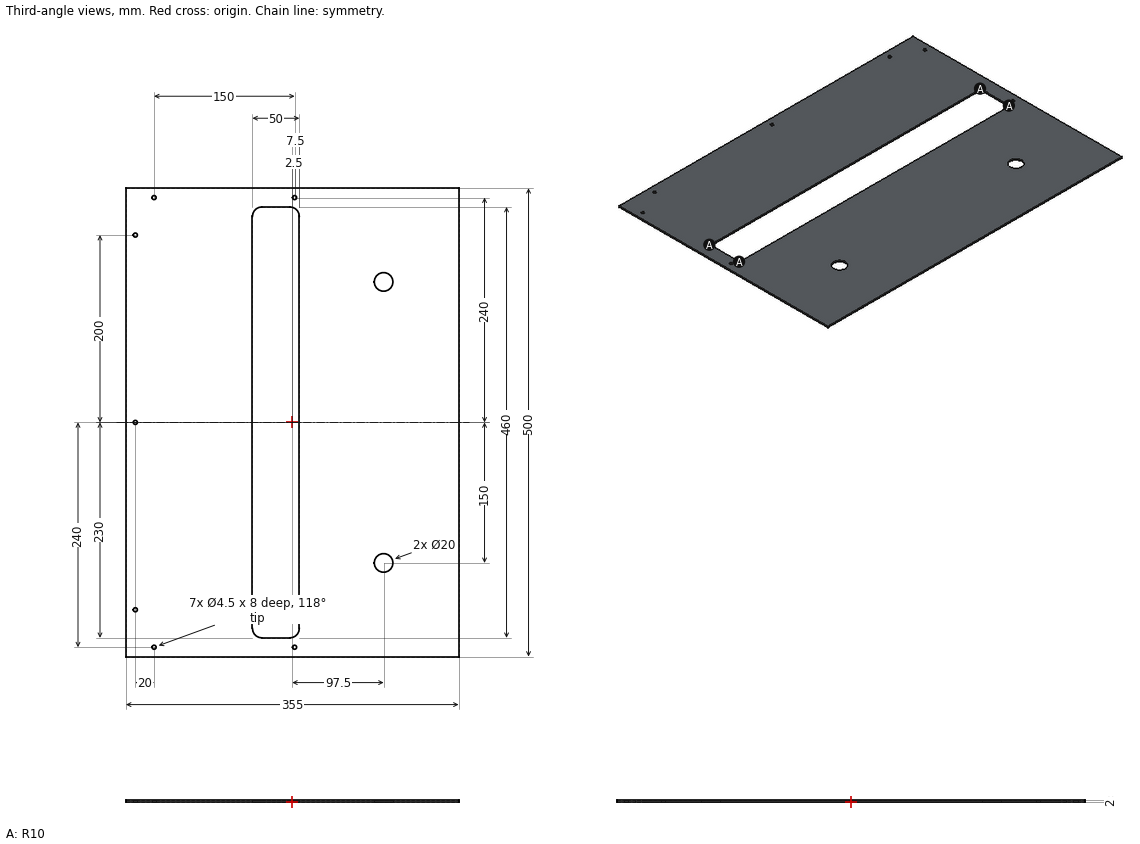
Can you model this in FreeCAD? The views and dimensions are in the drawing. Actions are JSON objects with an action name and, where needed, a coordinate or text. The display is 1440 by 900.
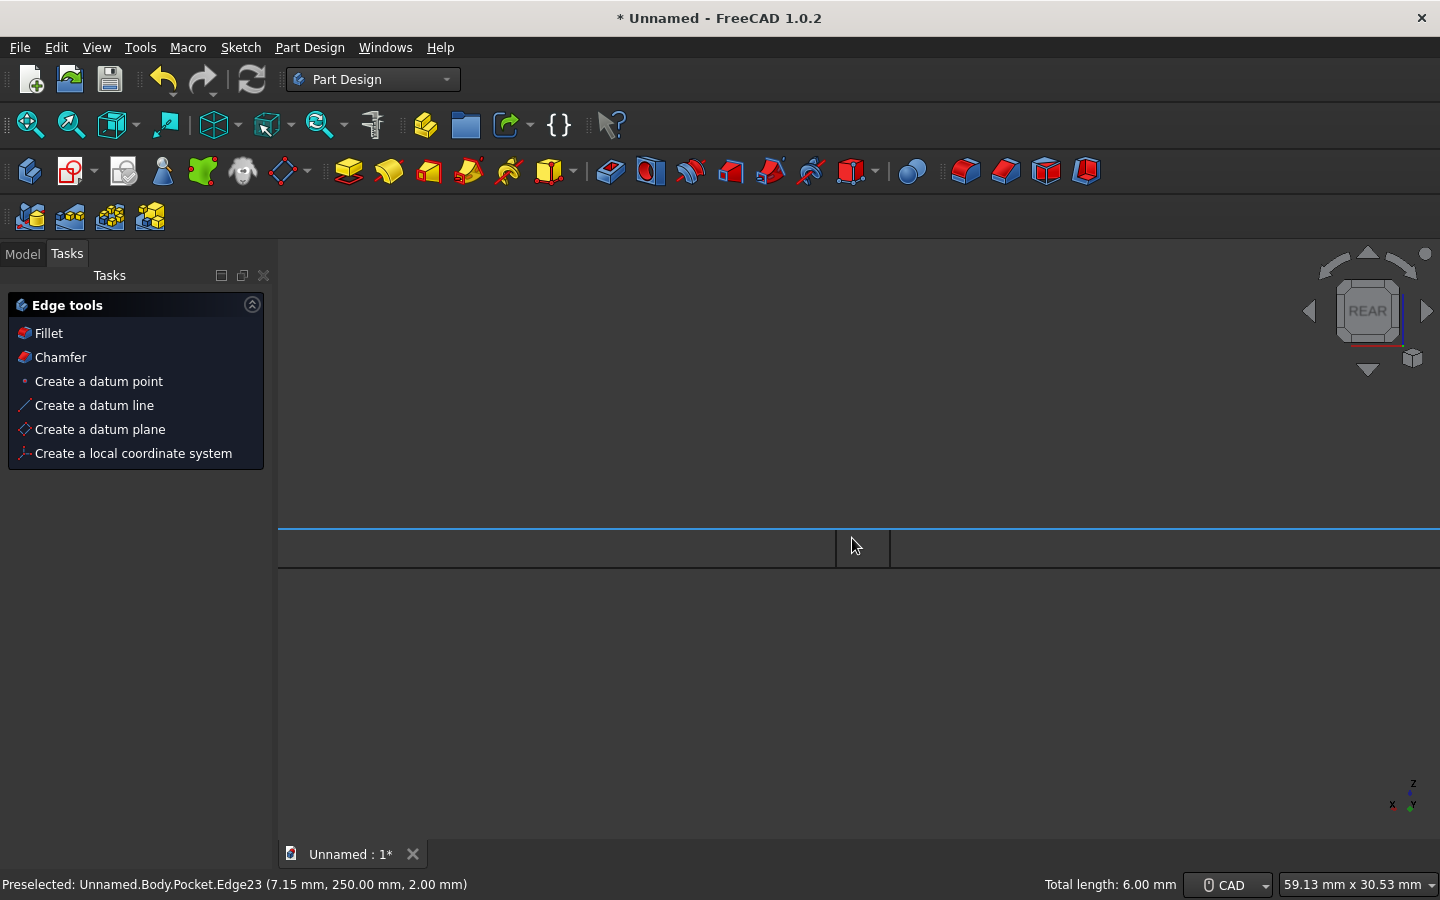
{"action": "left_click", "coordinate": [836, 548], "text": "ctrl"}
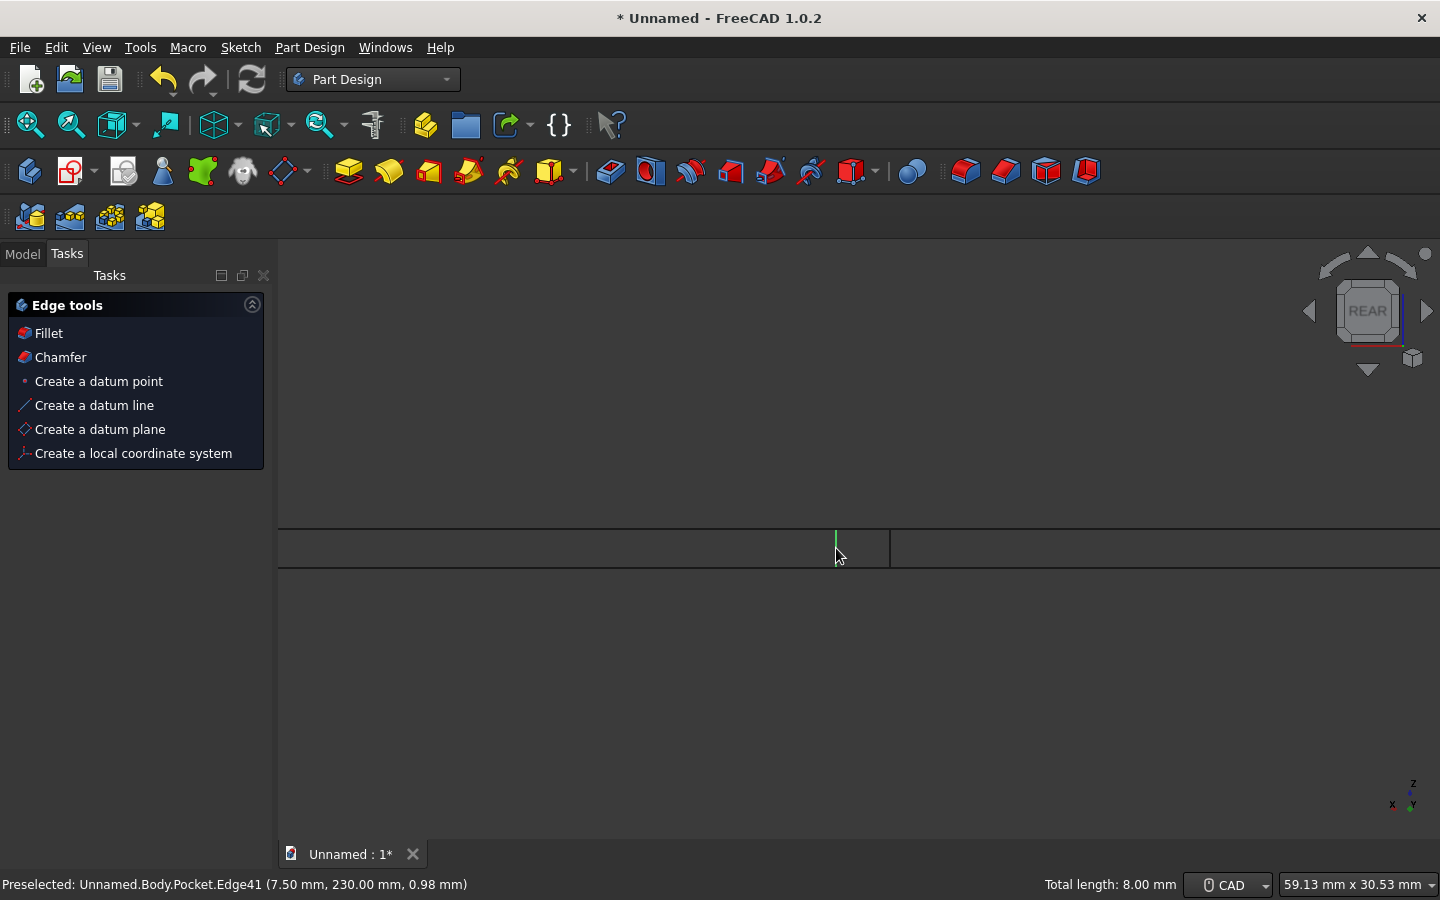
{"action": "key", "text": "v 1"}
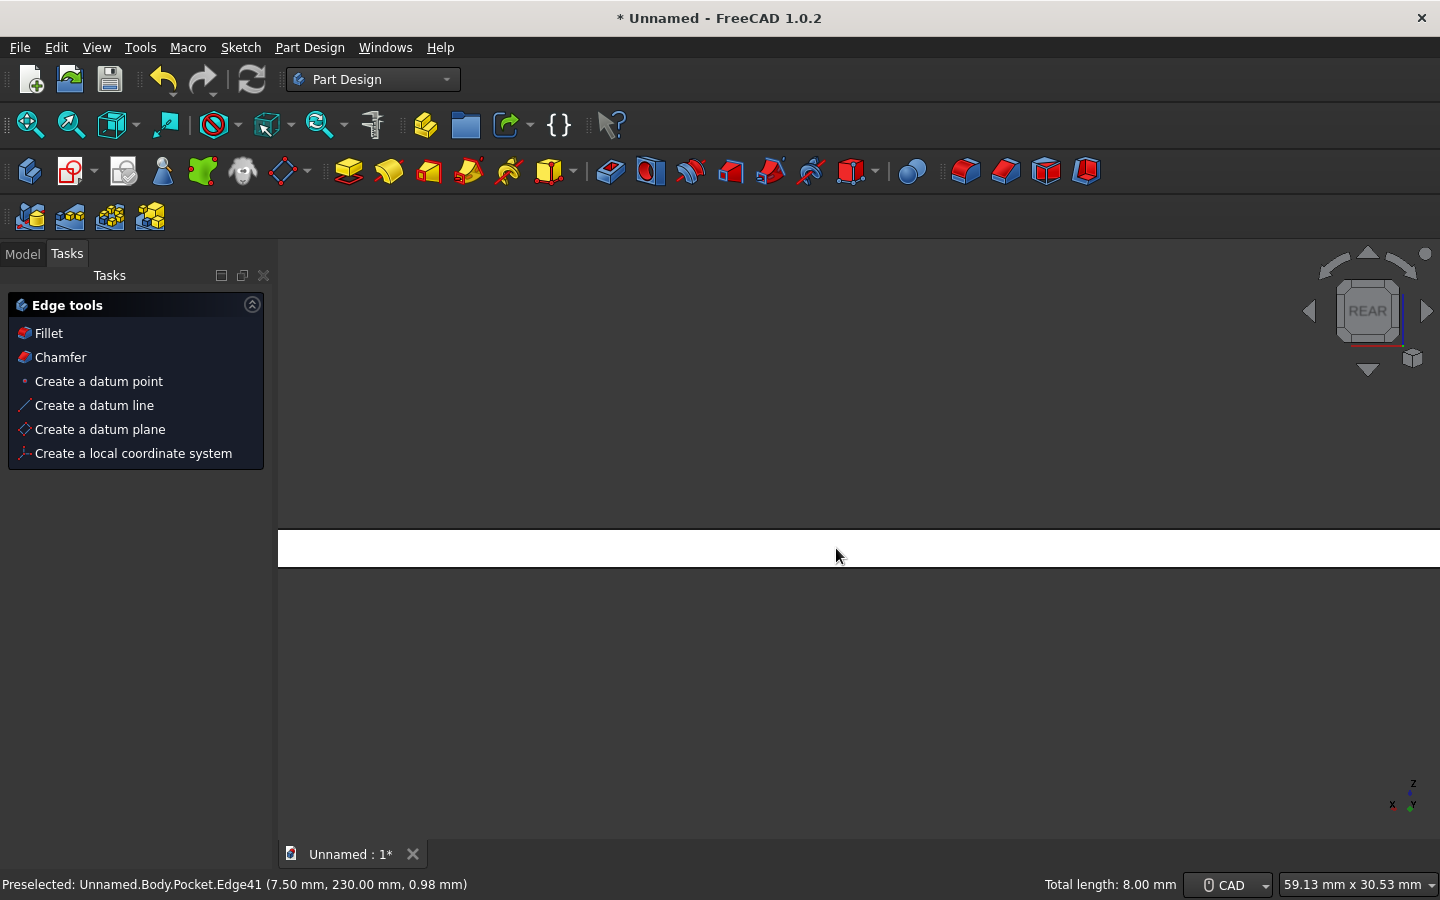
{"action": "left_click", "coordinate": [966, 172]}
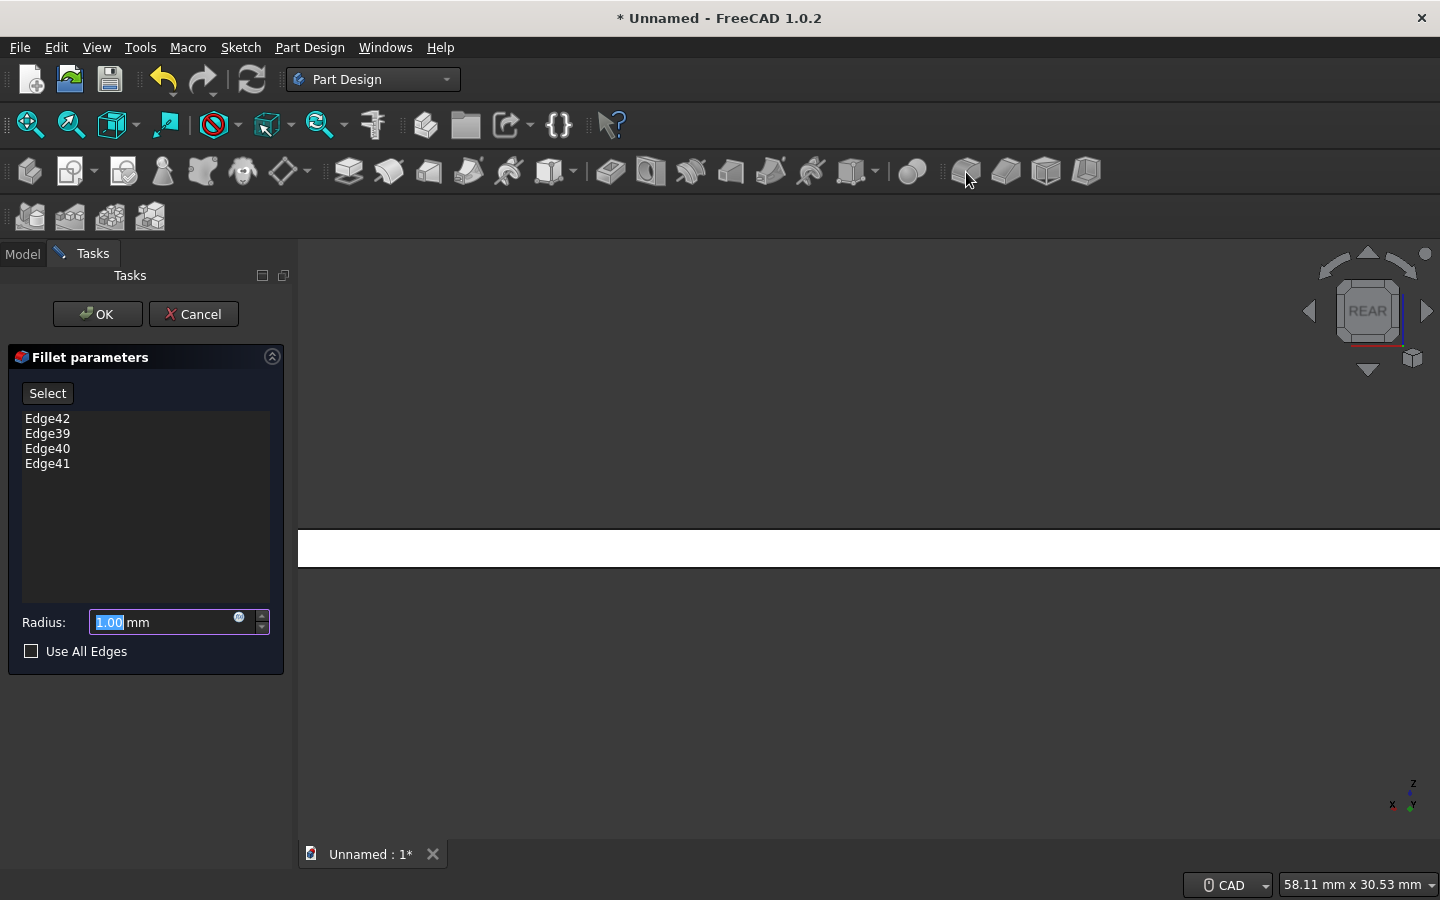
{"action": "type", "text": "10"}
{"action": "key", "text": "Tab"}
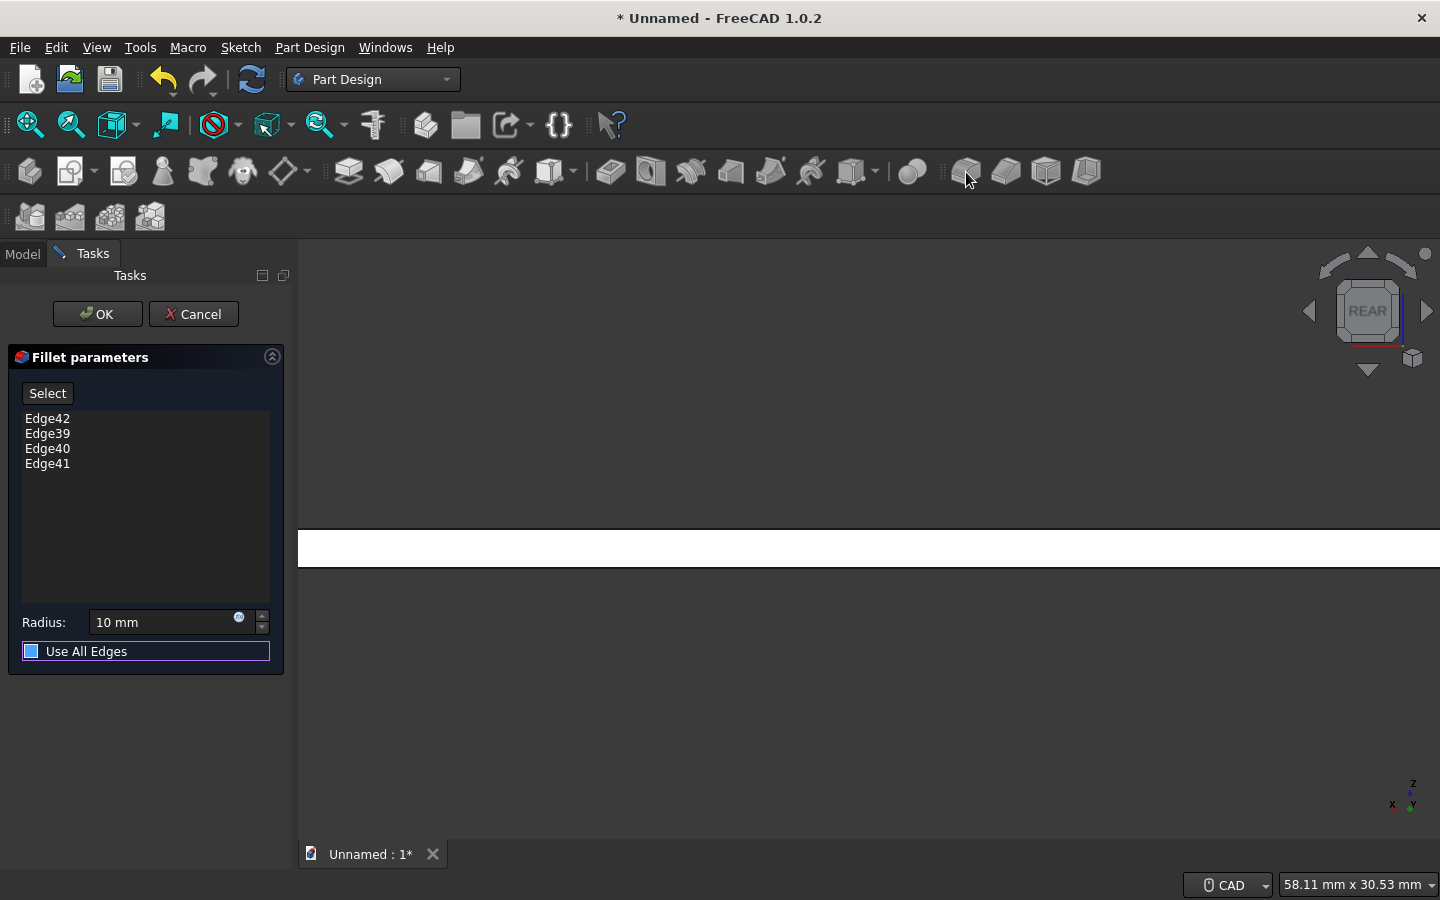
{"action": "left_click", "coordinate": [98, 314]}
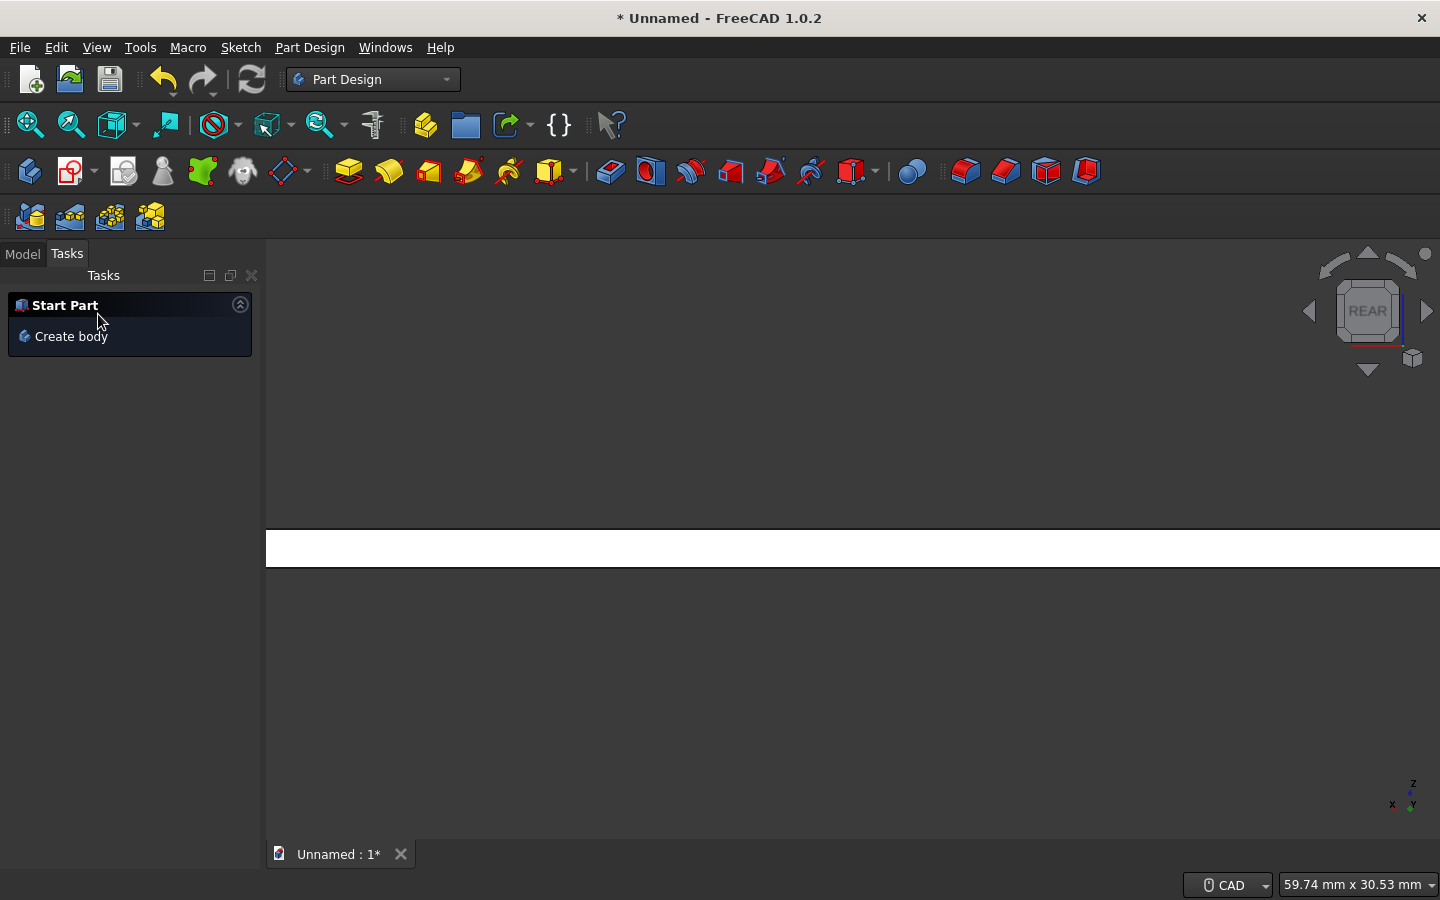
{"action": "left_click", "coordinate": [32, 126]}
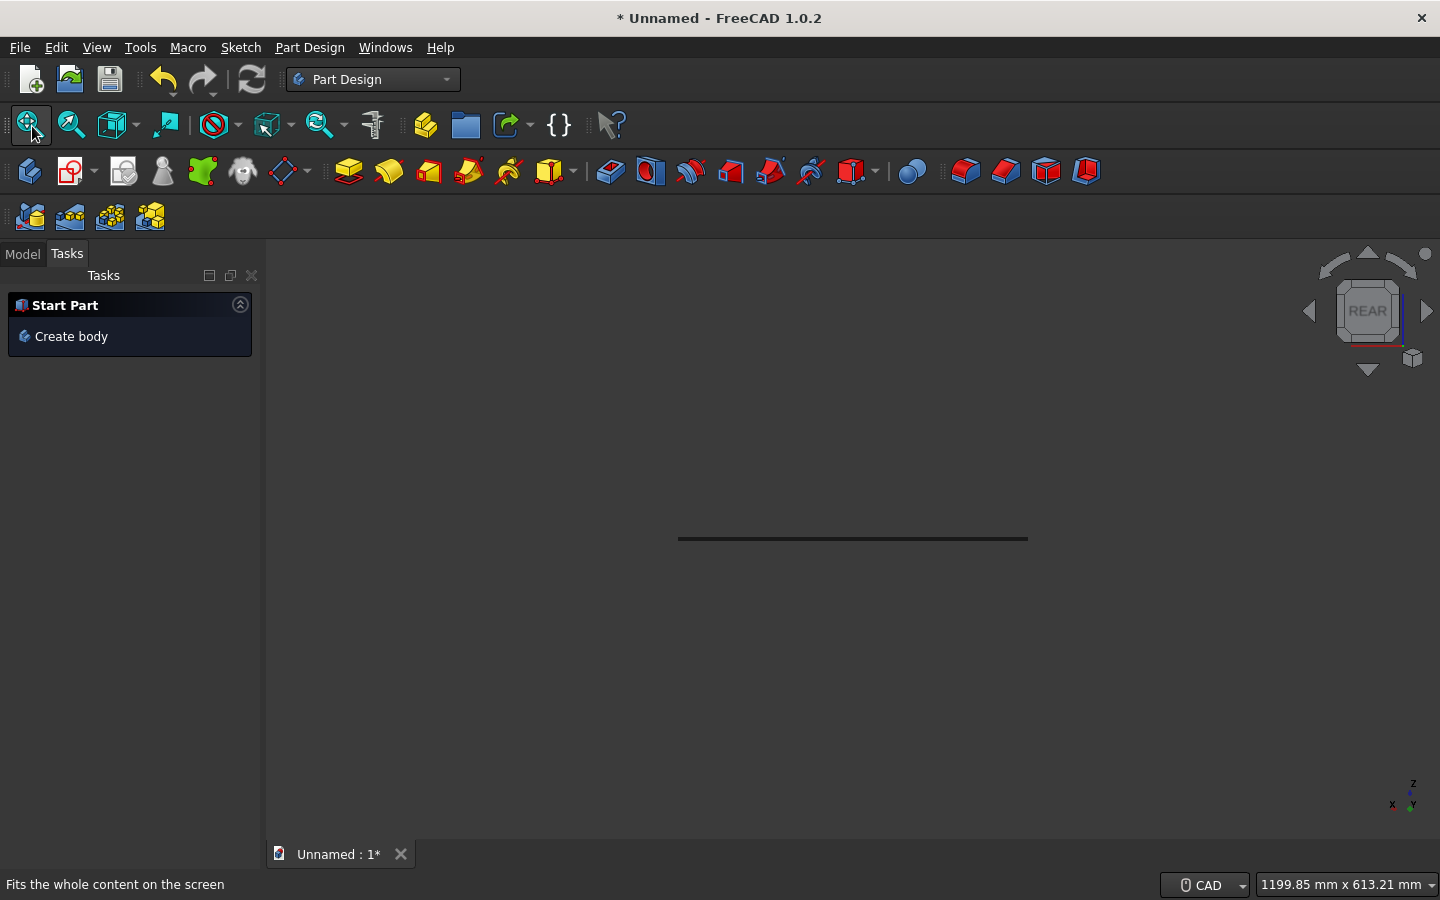
{"action": "left_click", "coordinate": [70, 172]}